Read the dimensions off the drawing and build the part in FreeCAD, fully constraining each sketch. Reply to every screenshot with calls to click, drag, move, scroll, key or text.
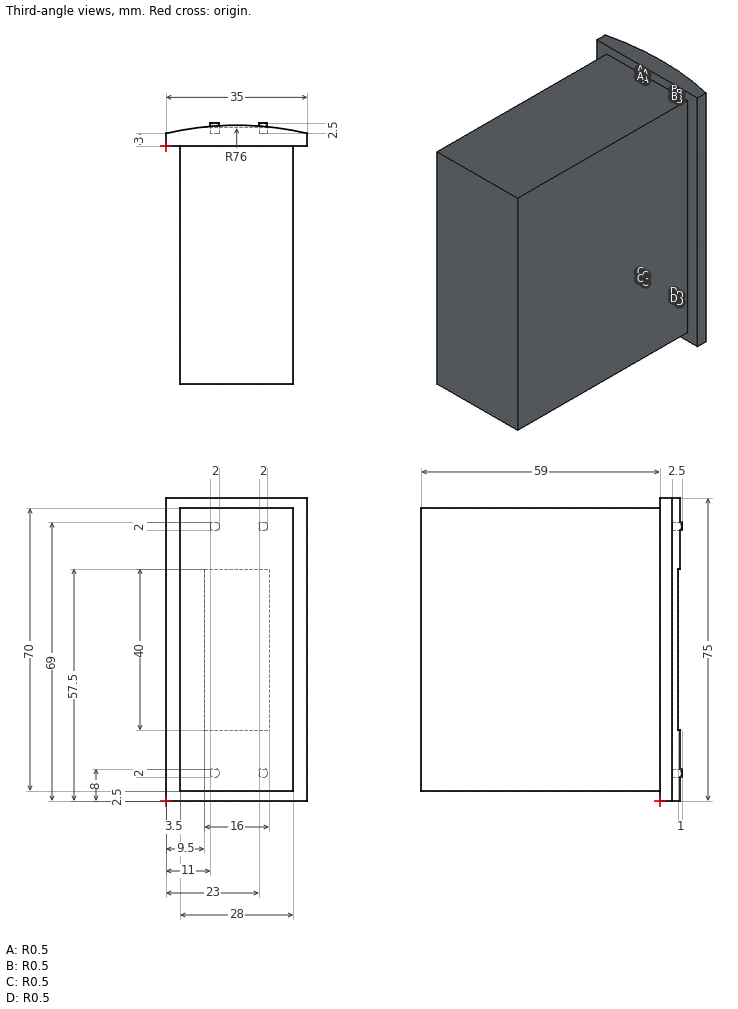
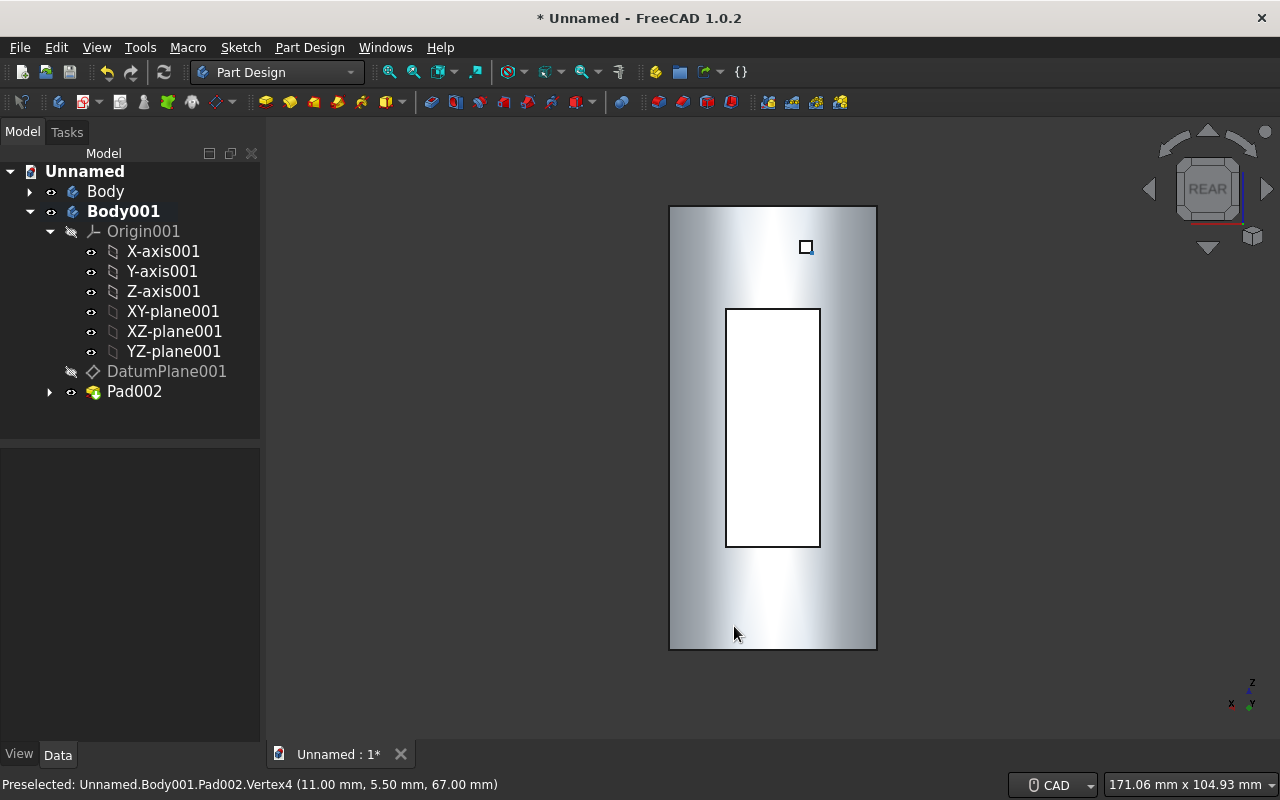
scroll(812, 240, up, 5)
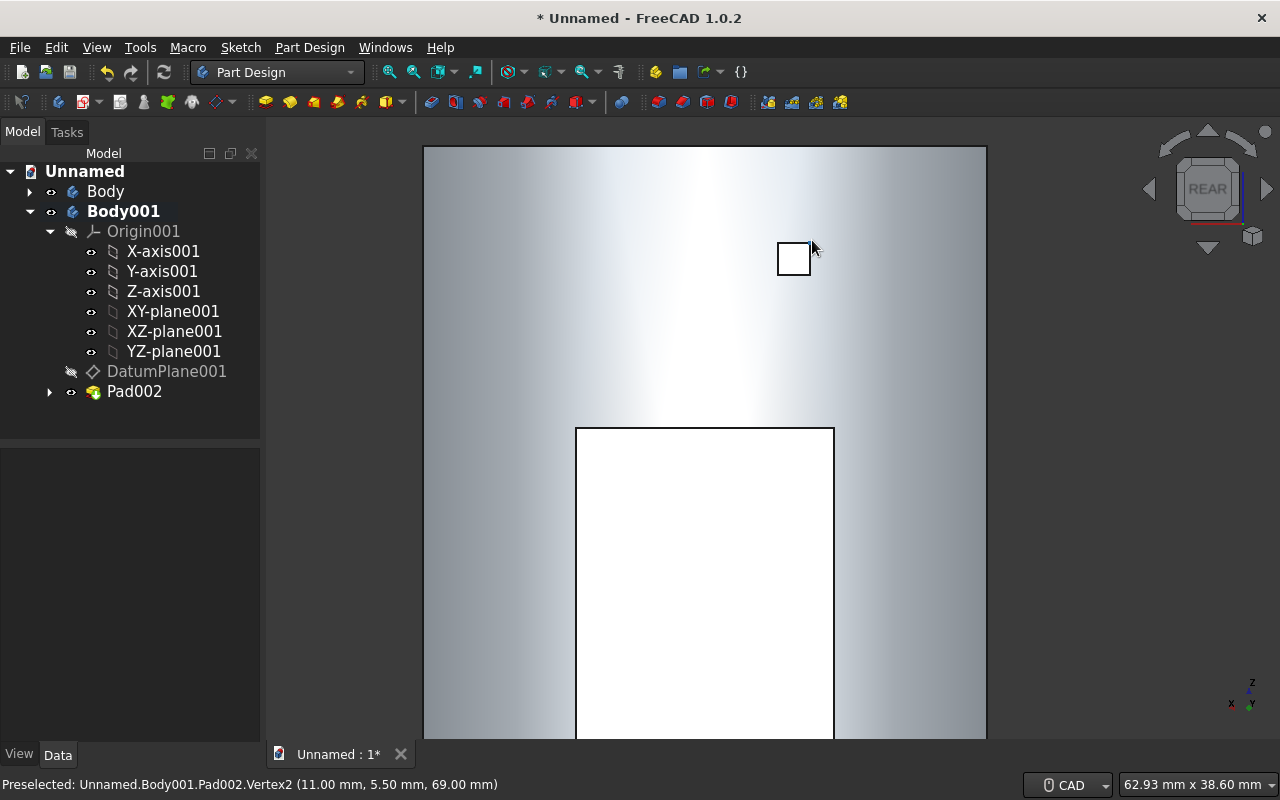
key(v)
key(f)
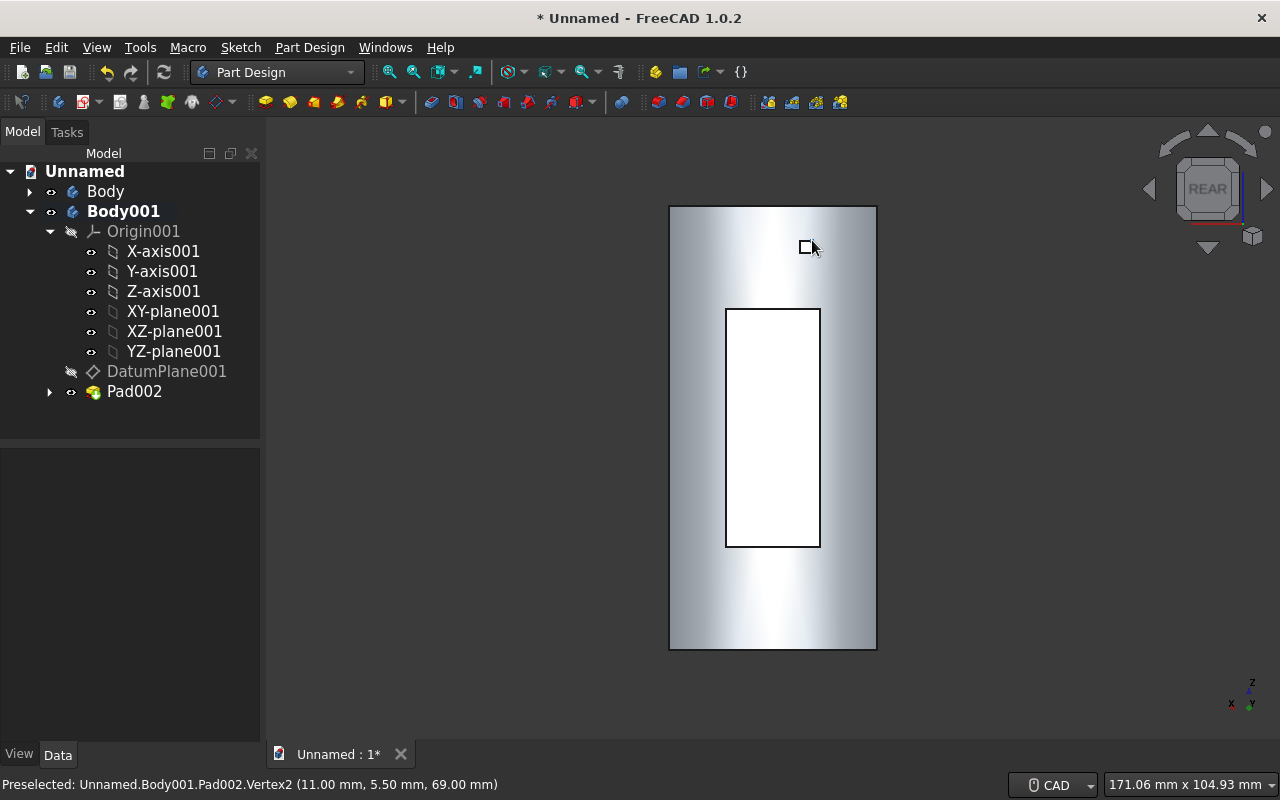
key(6)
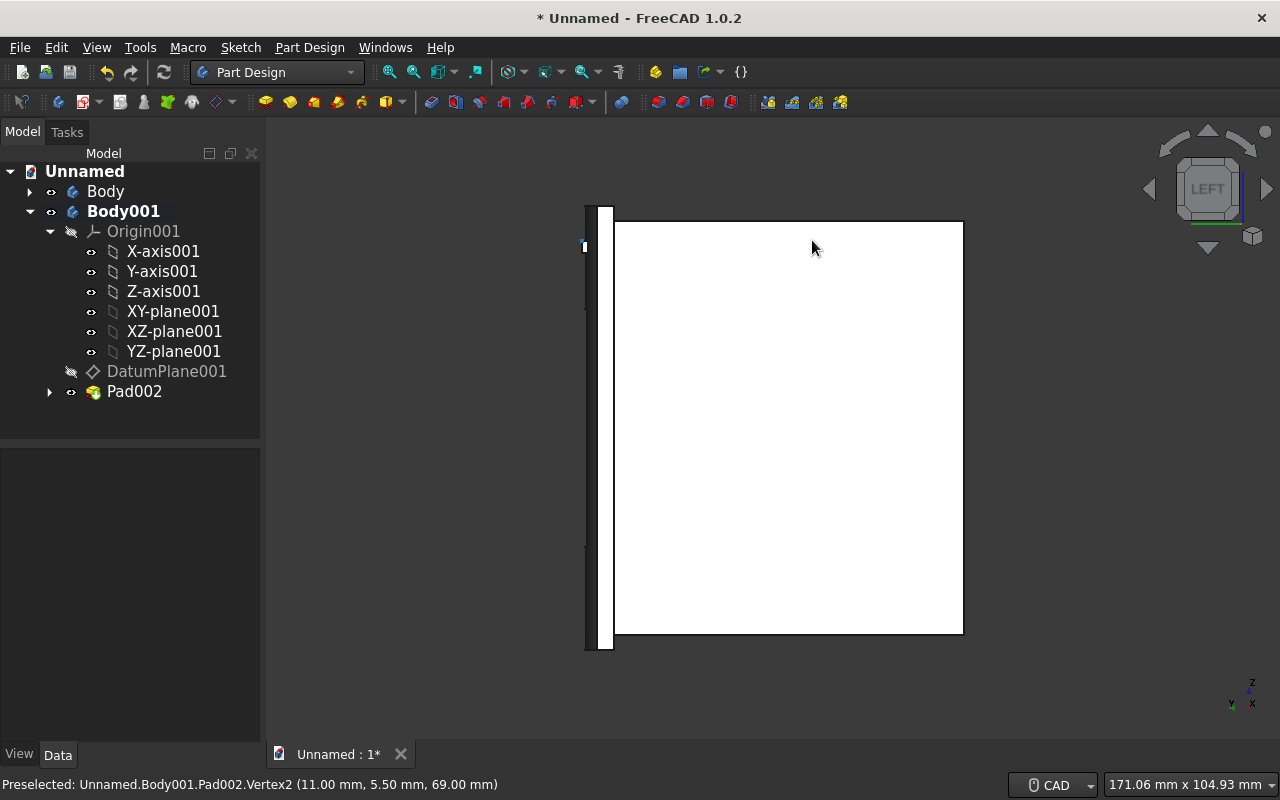
key(v)
key(f)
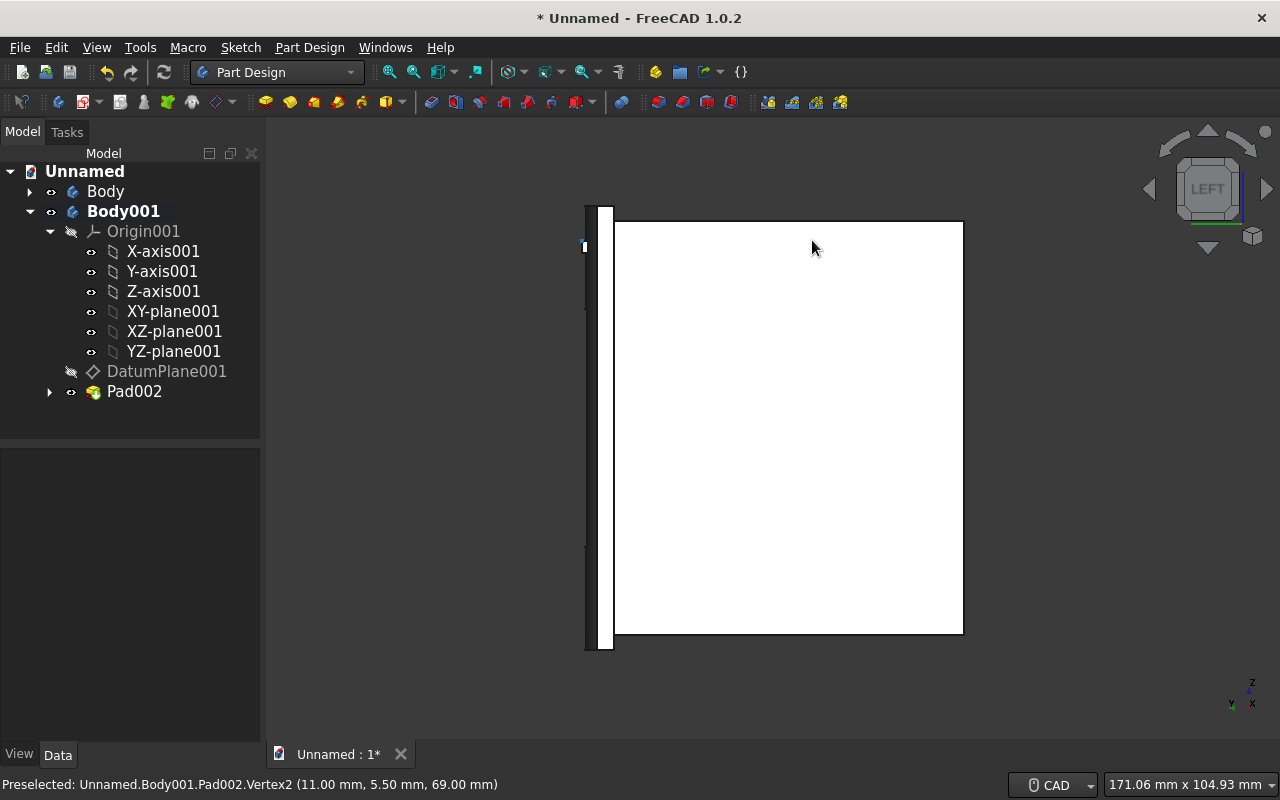
scroll(589, 240, up, 5)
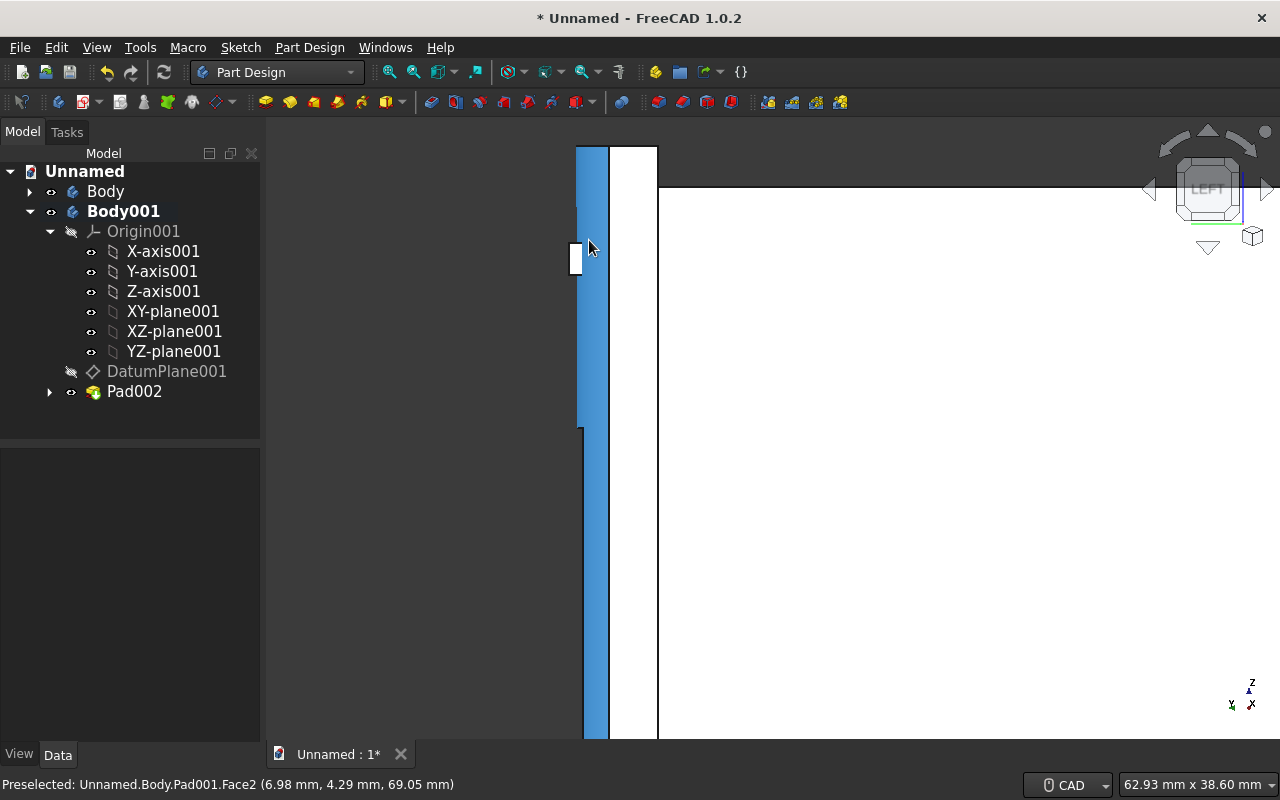
click(577, 242)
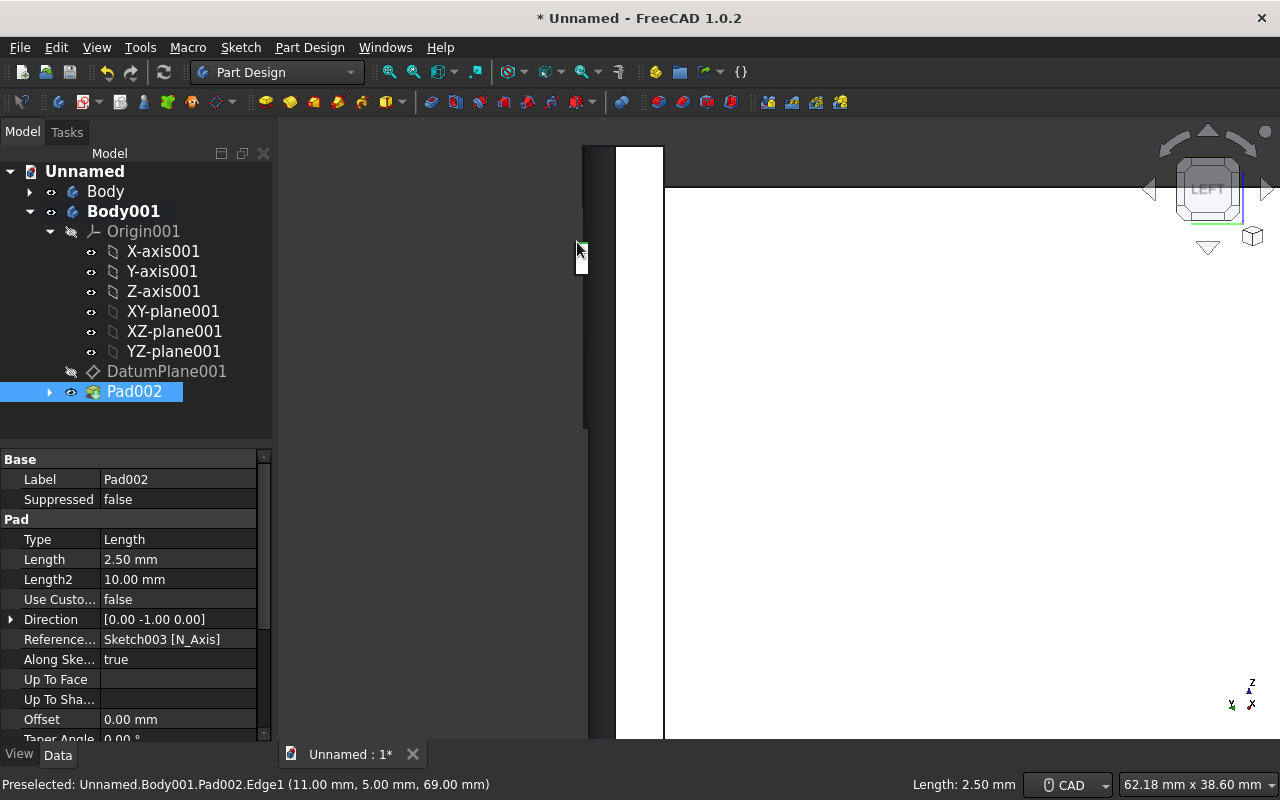
click(583, 274, ctrl)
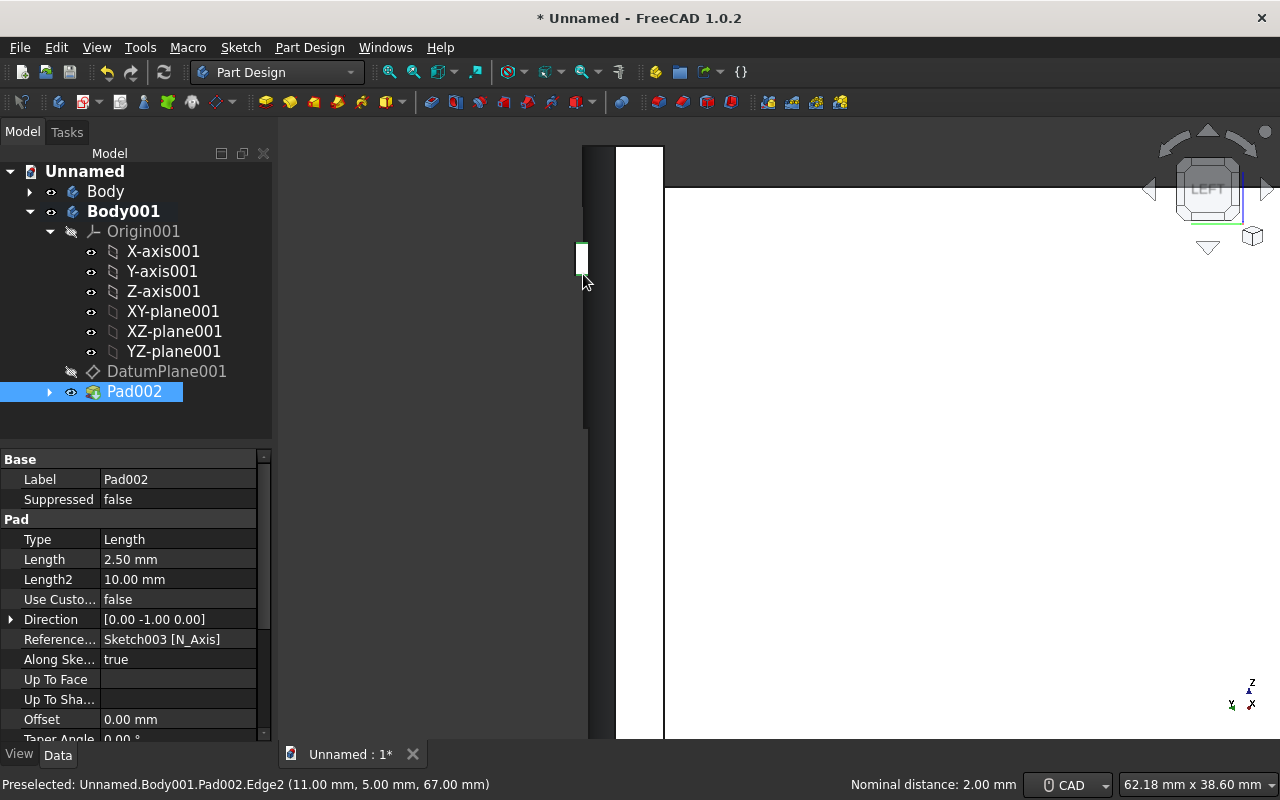
key(v)
key(f)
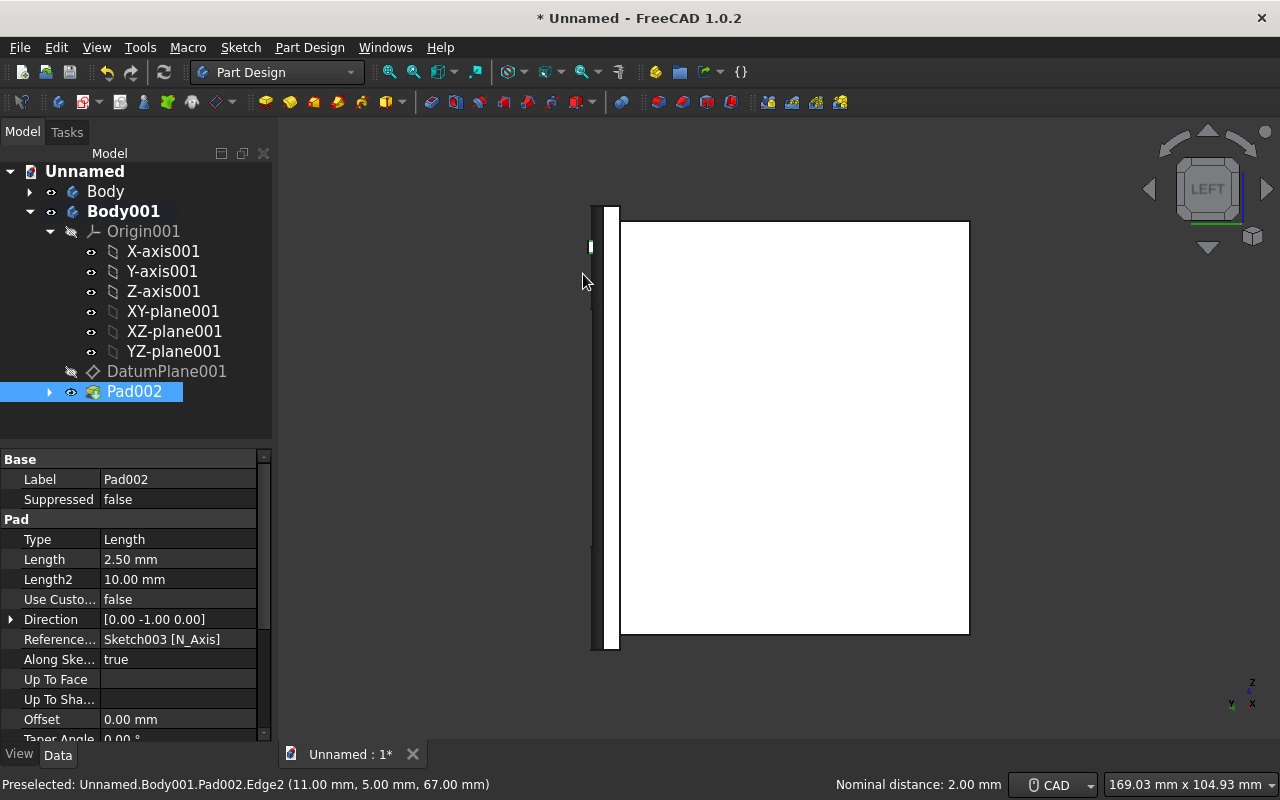
key(v)
key(3)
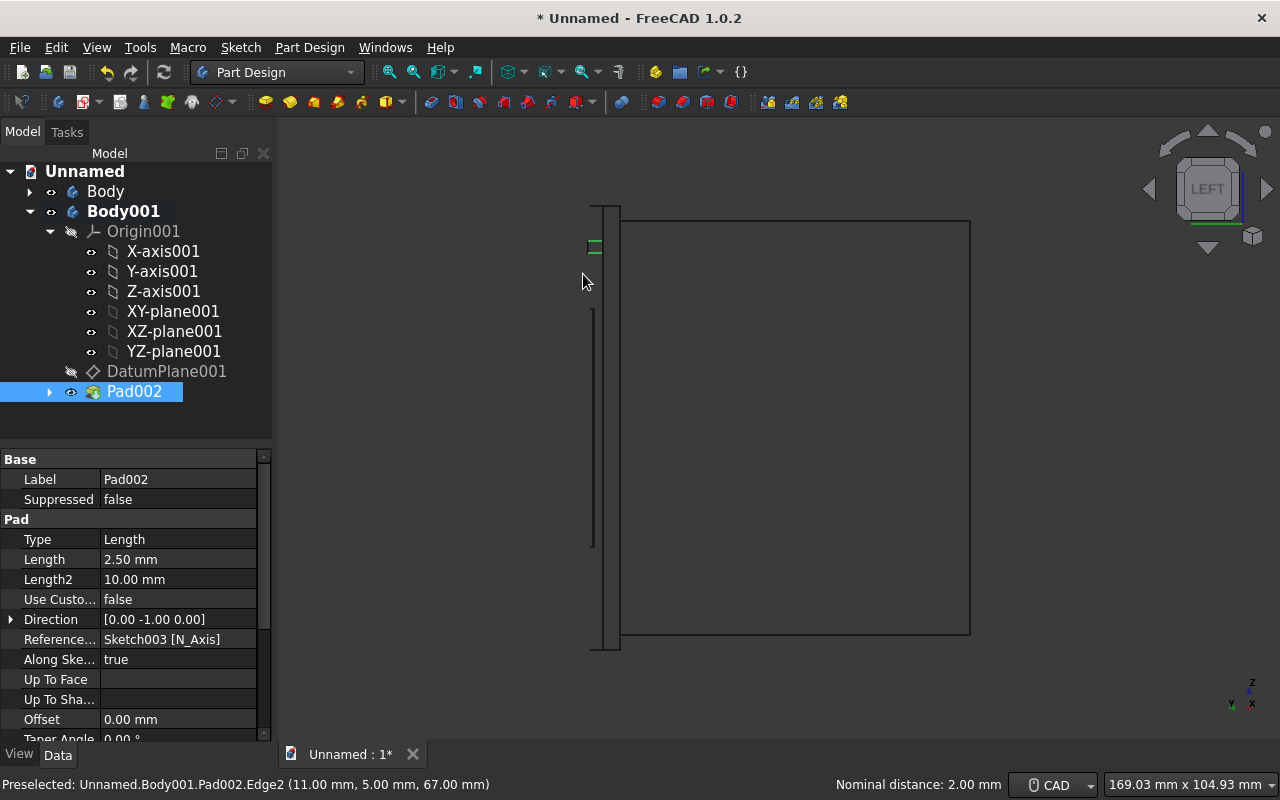
key(0)